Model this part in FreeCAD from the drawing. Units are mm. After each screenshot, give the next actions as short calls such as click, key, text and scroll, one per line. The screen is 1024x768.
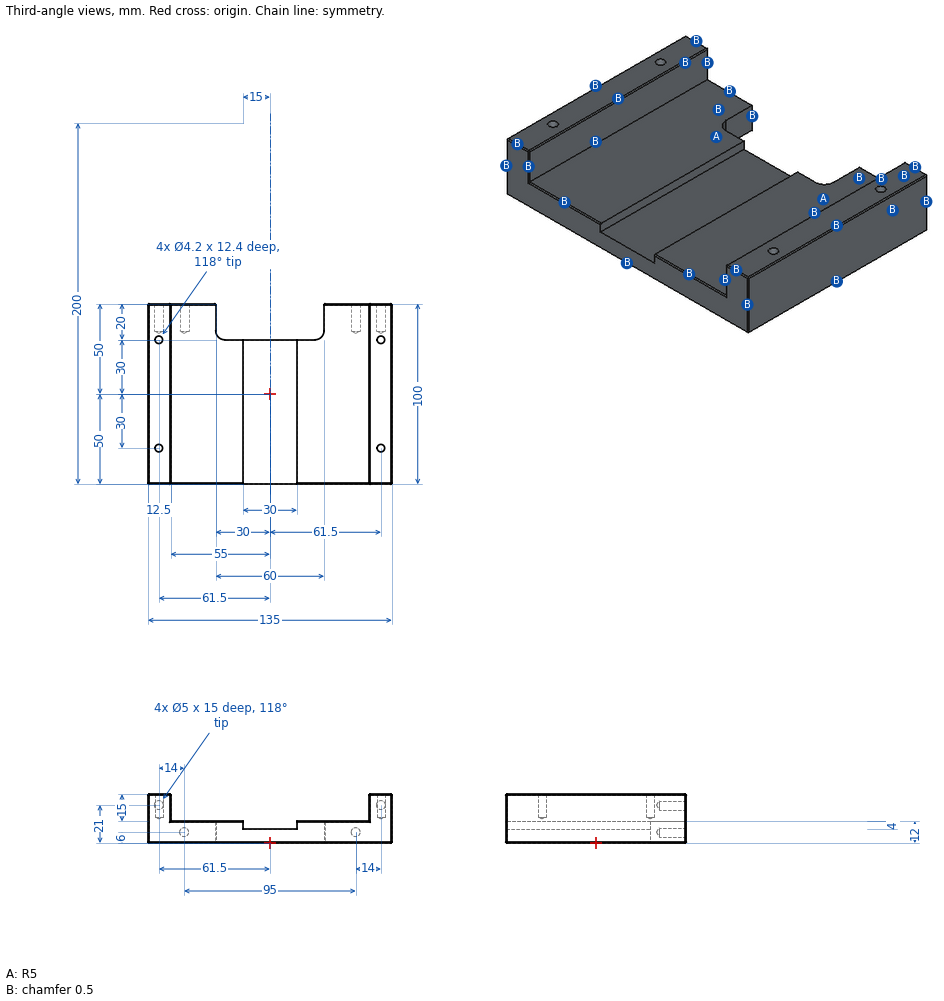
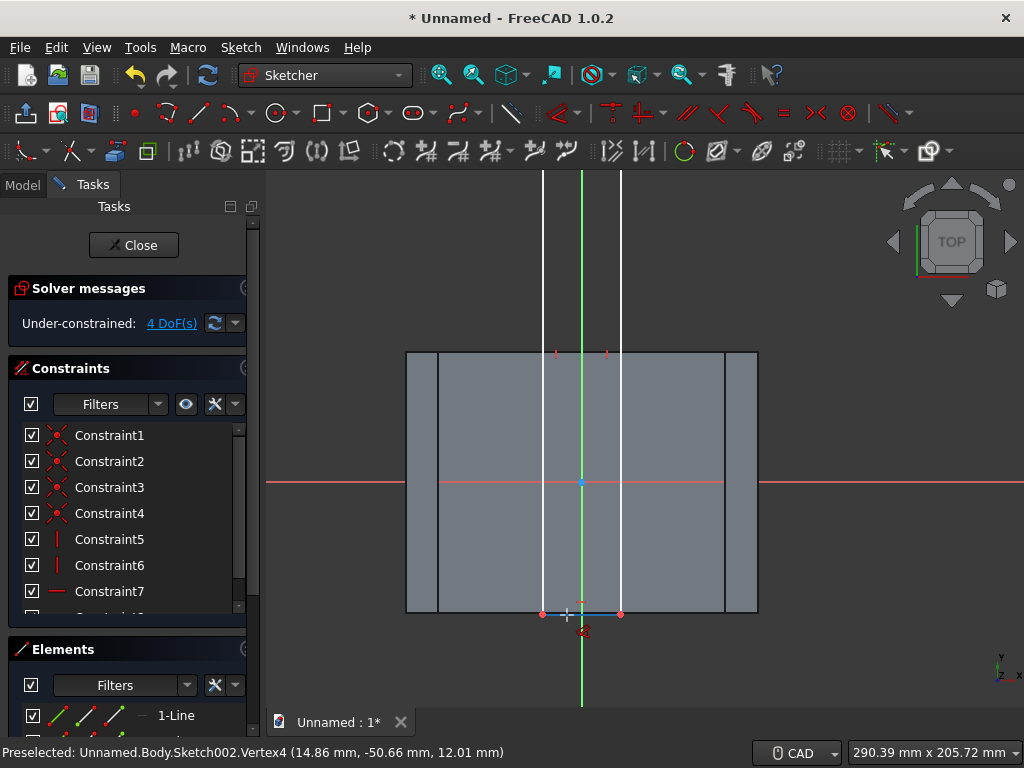
click(566, 615)
click(564, 649)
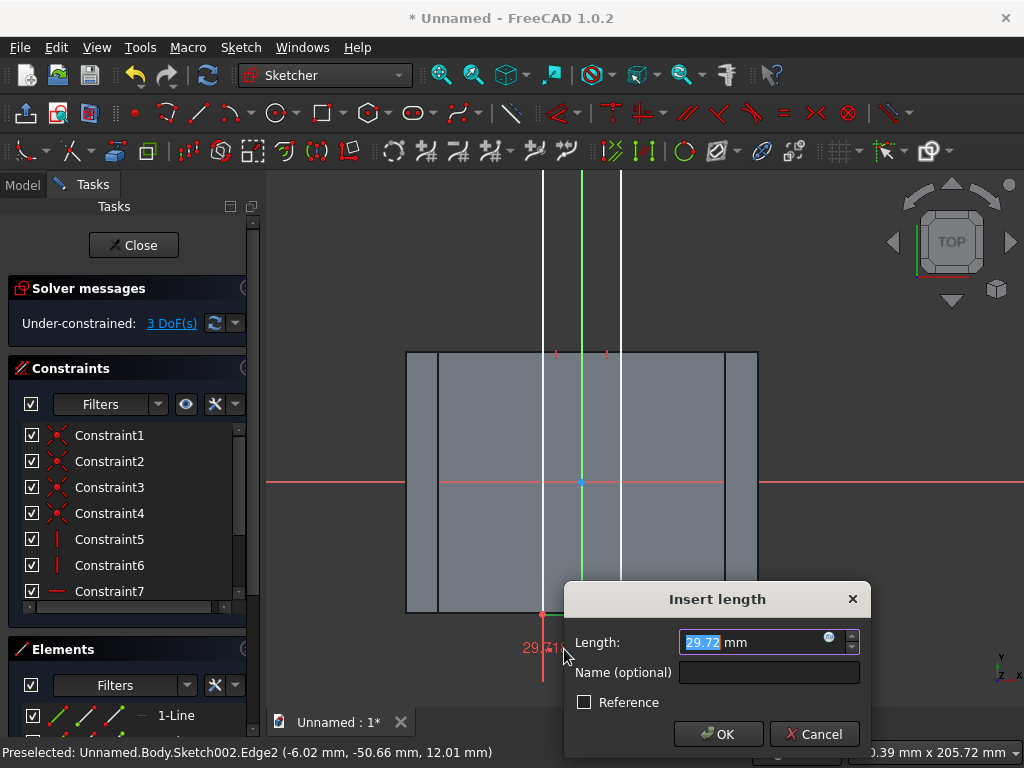
text(30)
key(Return)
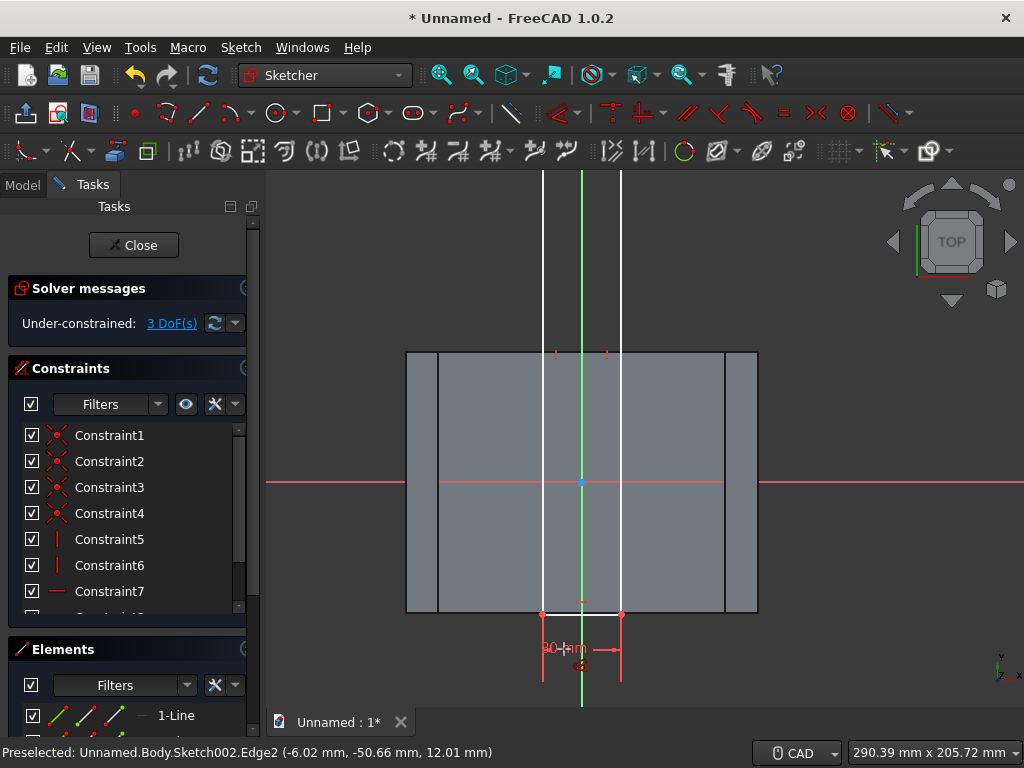
click(543, 249)
click(509, 406)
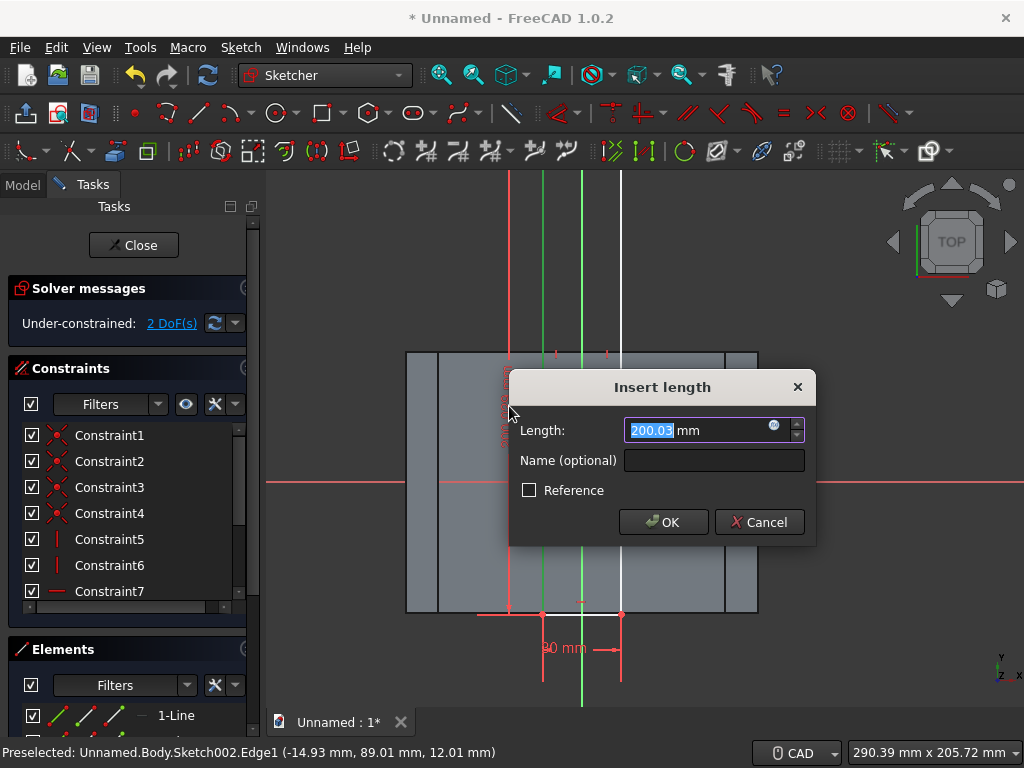
text(200)
key(Return)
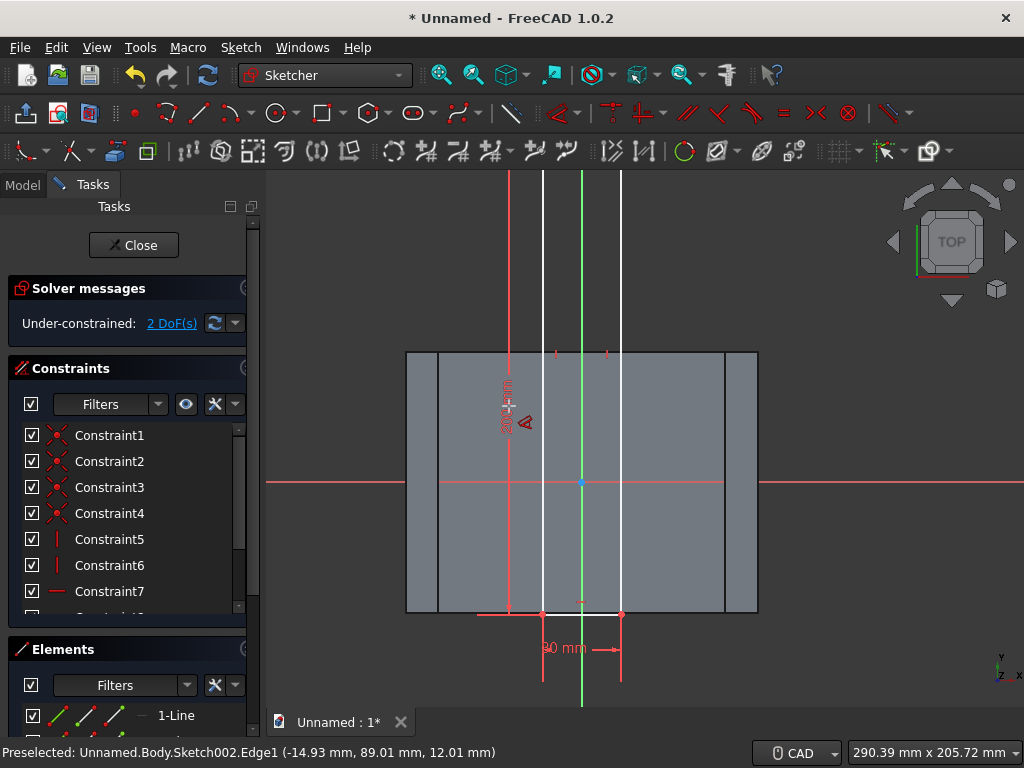
scroll(566, 615, down, 2)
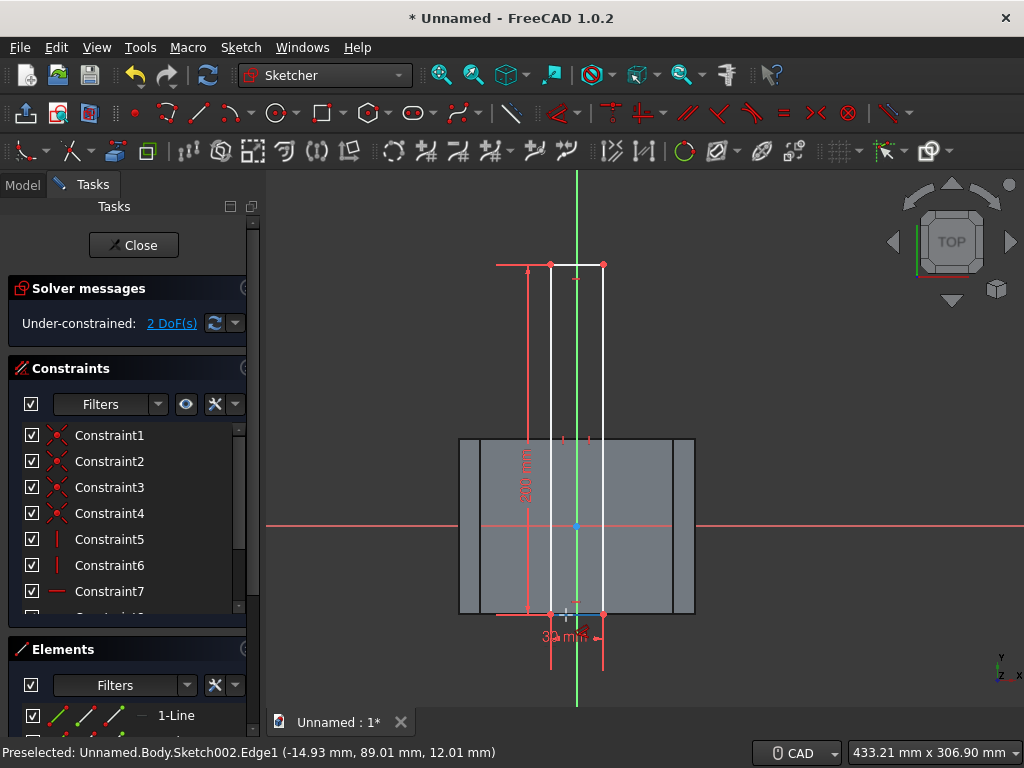
scroll(551, 265, up, 3)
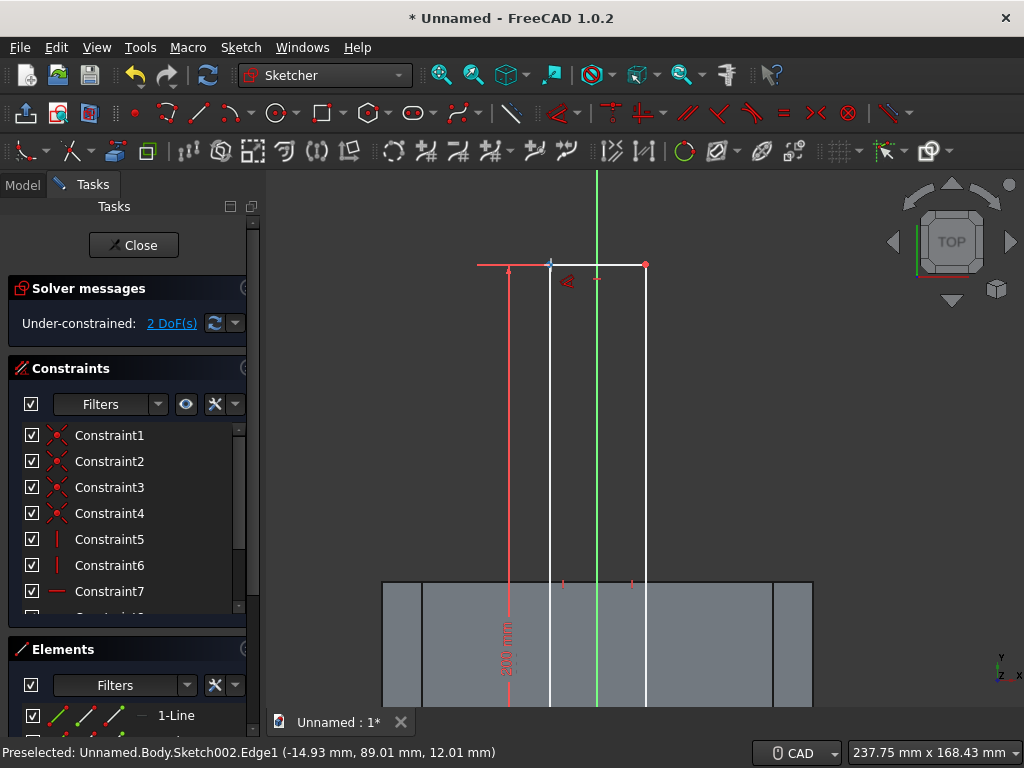
click(550, 265)
click(574, 231)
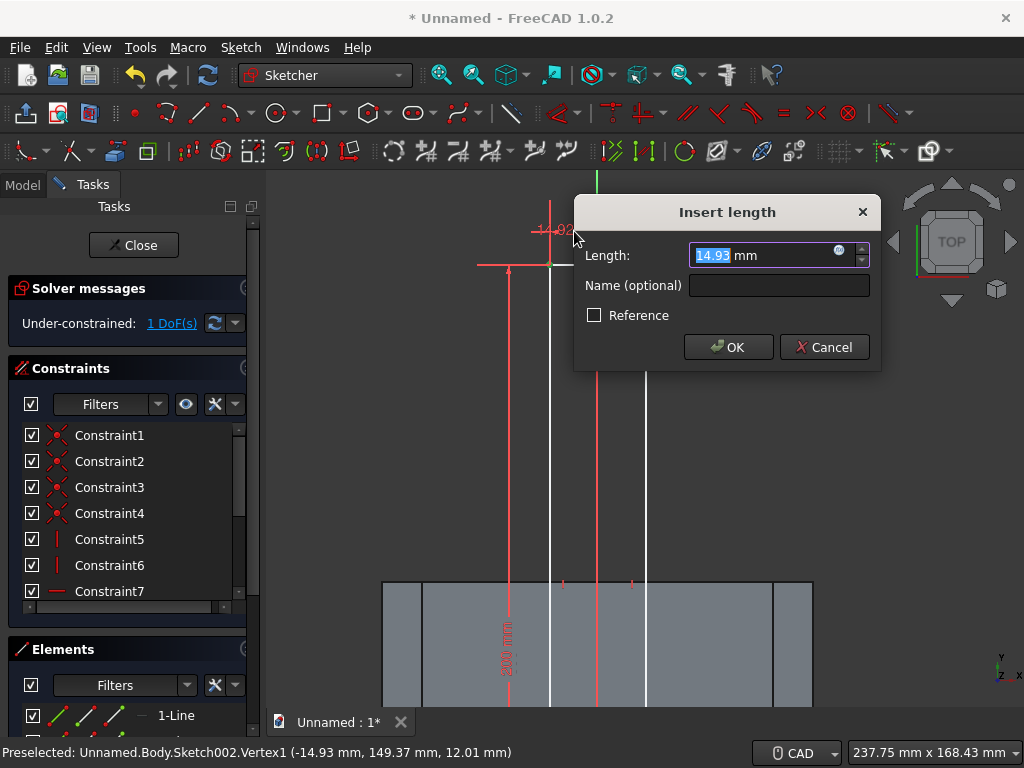
text(15)
key(Return)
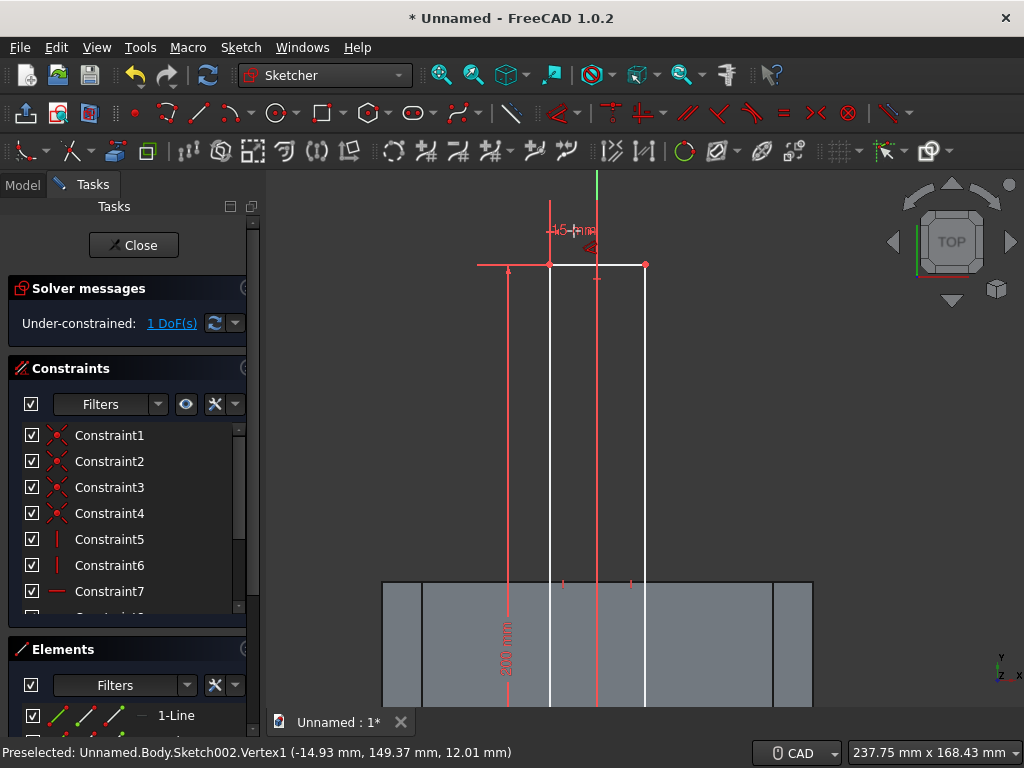
scroll(551, 264, down, 3)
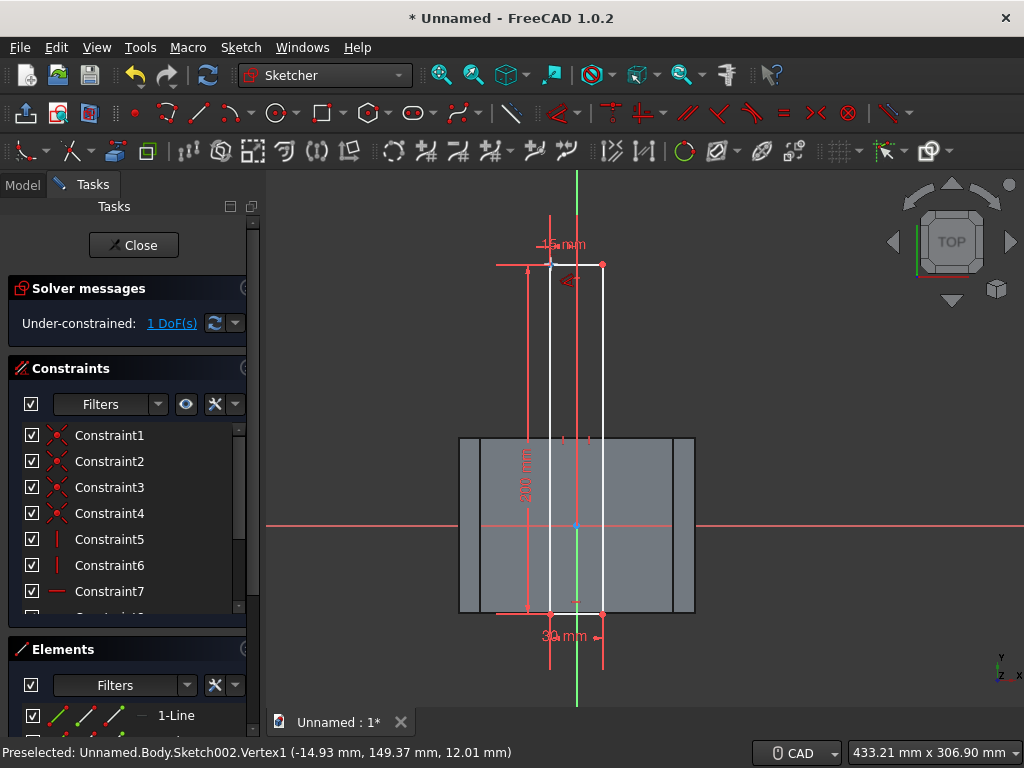
click(550, 614)
click(516, 570)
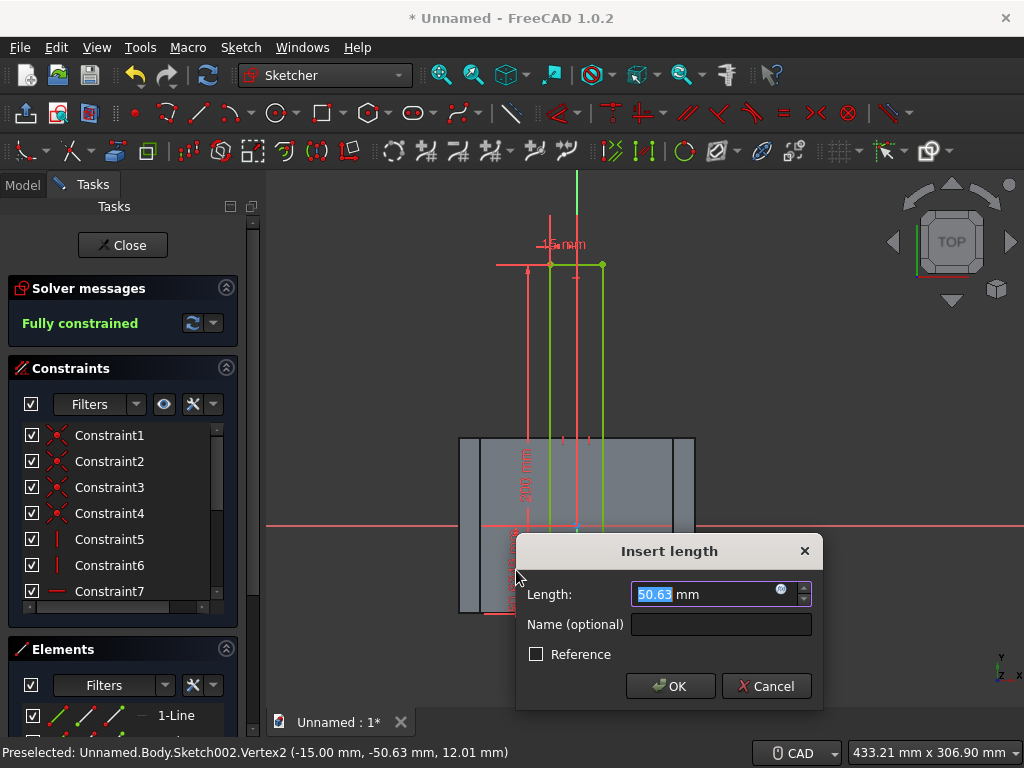
text(50)
key(Return)
key(Escape)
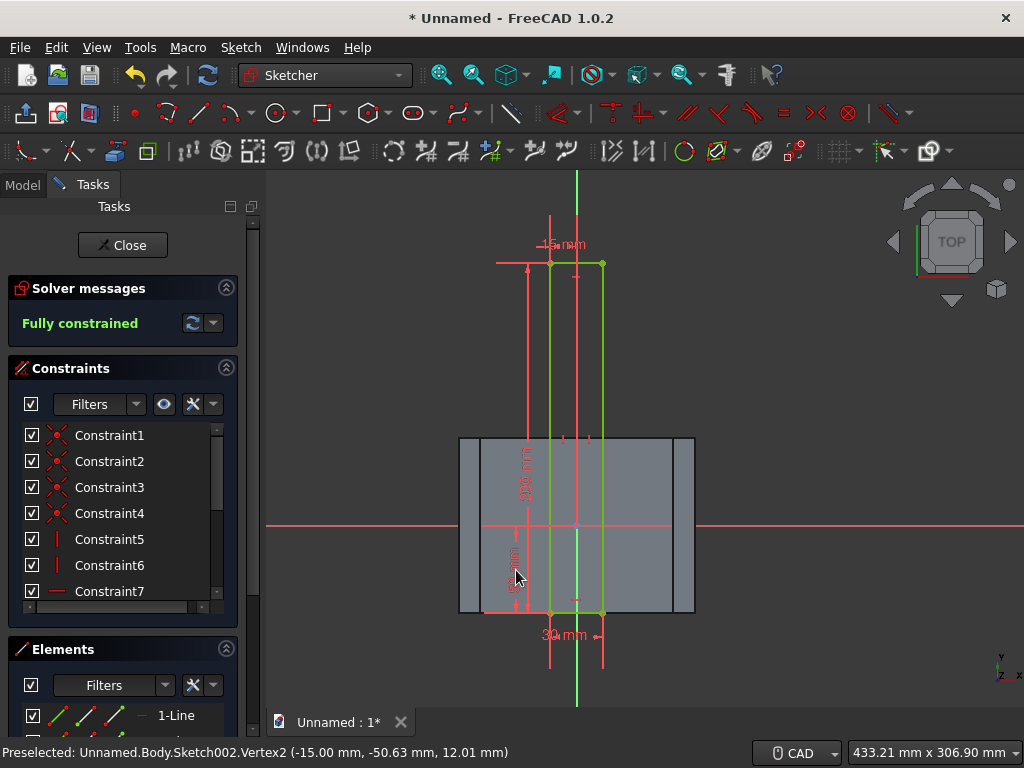
click(123, 245)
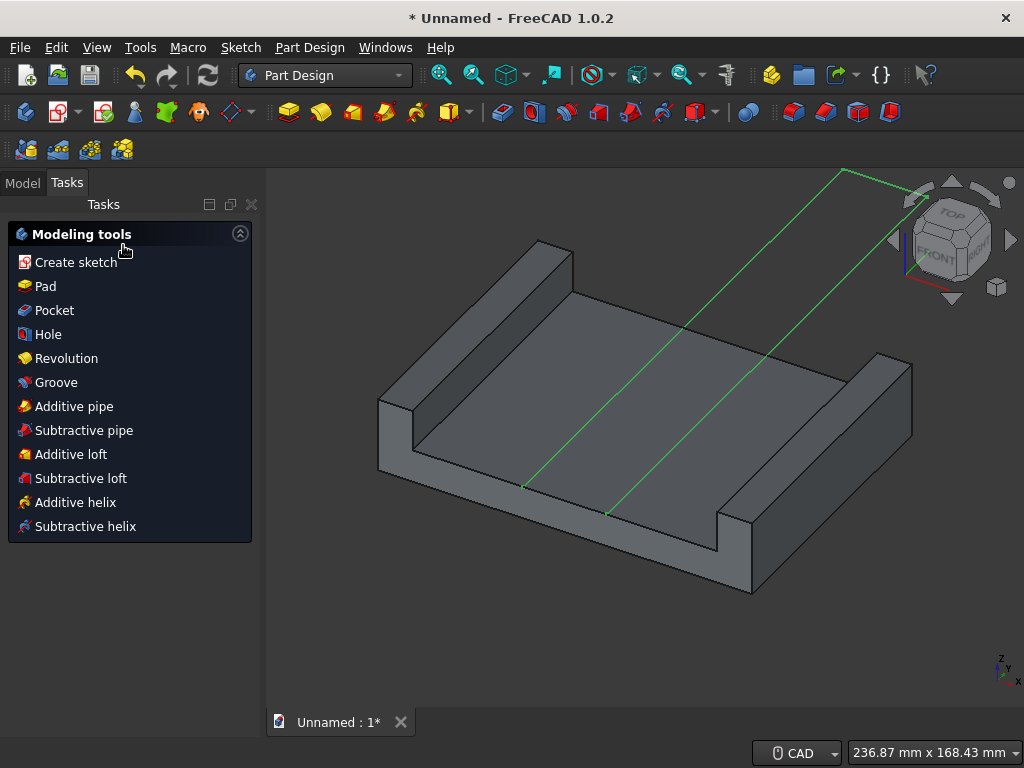
click(504, 112)